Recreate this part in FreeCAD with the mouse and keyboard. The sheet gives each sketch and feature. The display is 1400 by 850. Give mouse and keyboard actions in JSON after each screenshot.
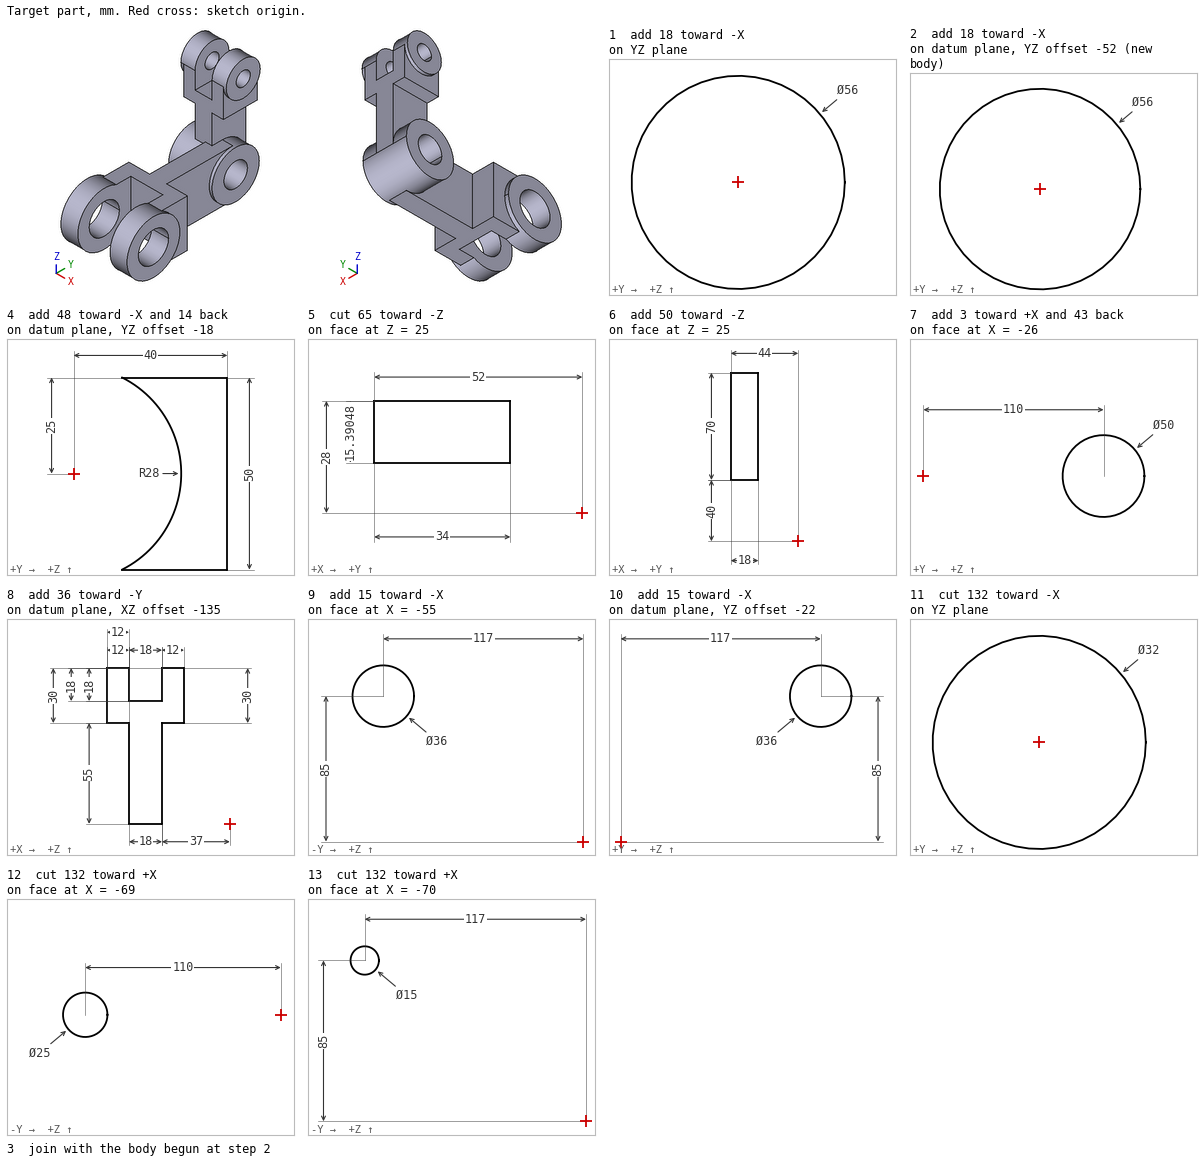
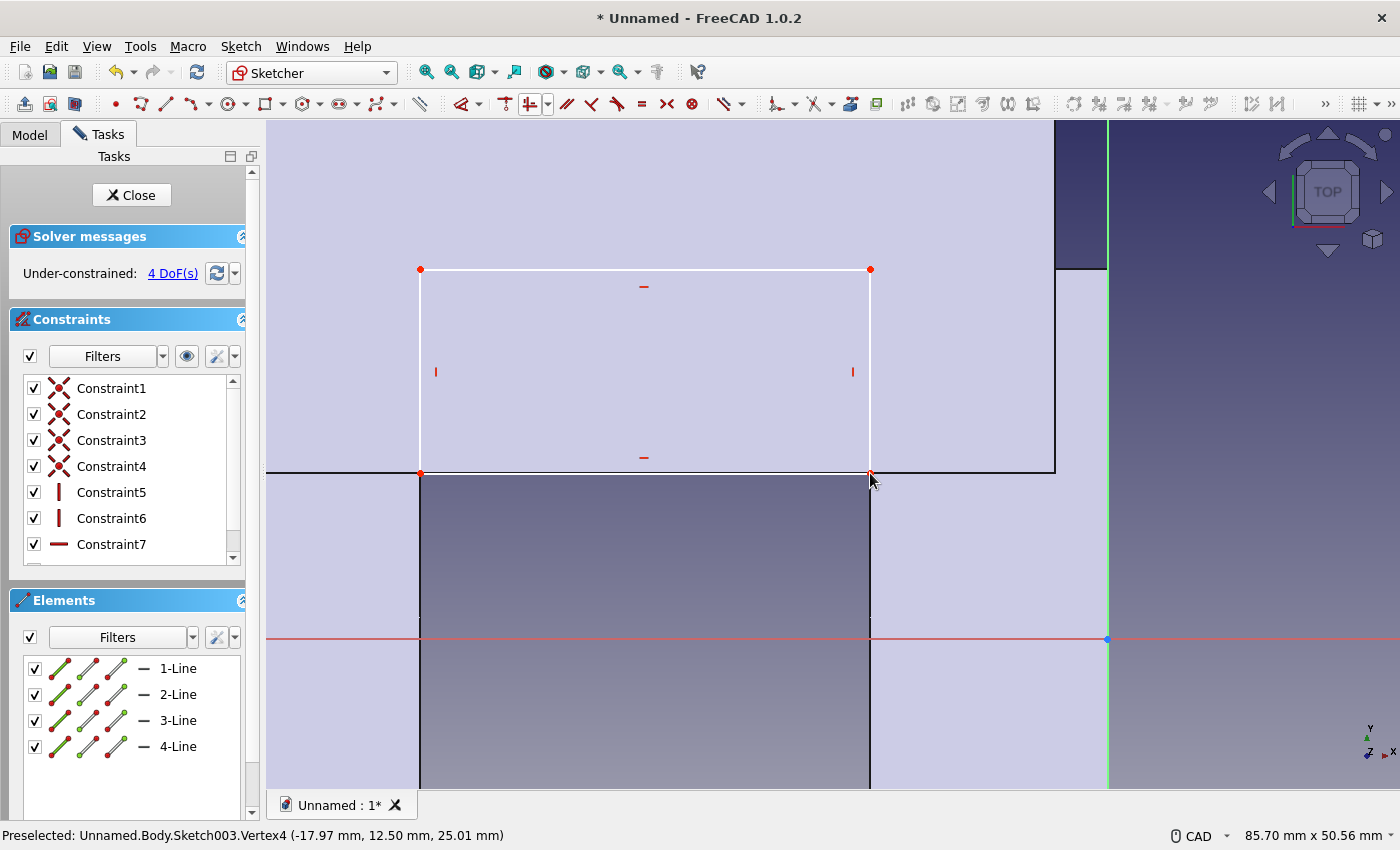
{"action": "left_click", "coordinate": [555, 474]}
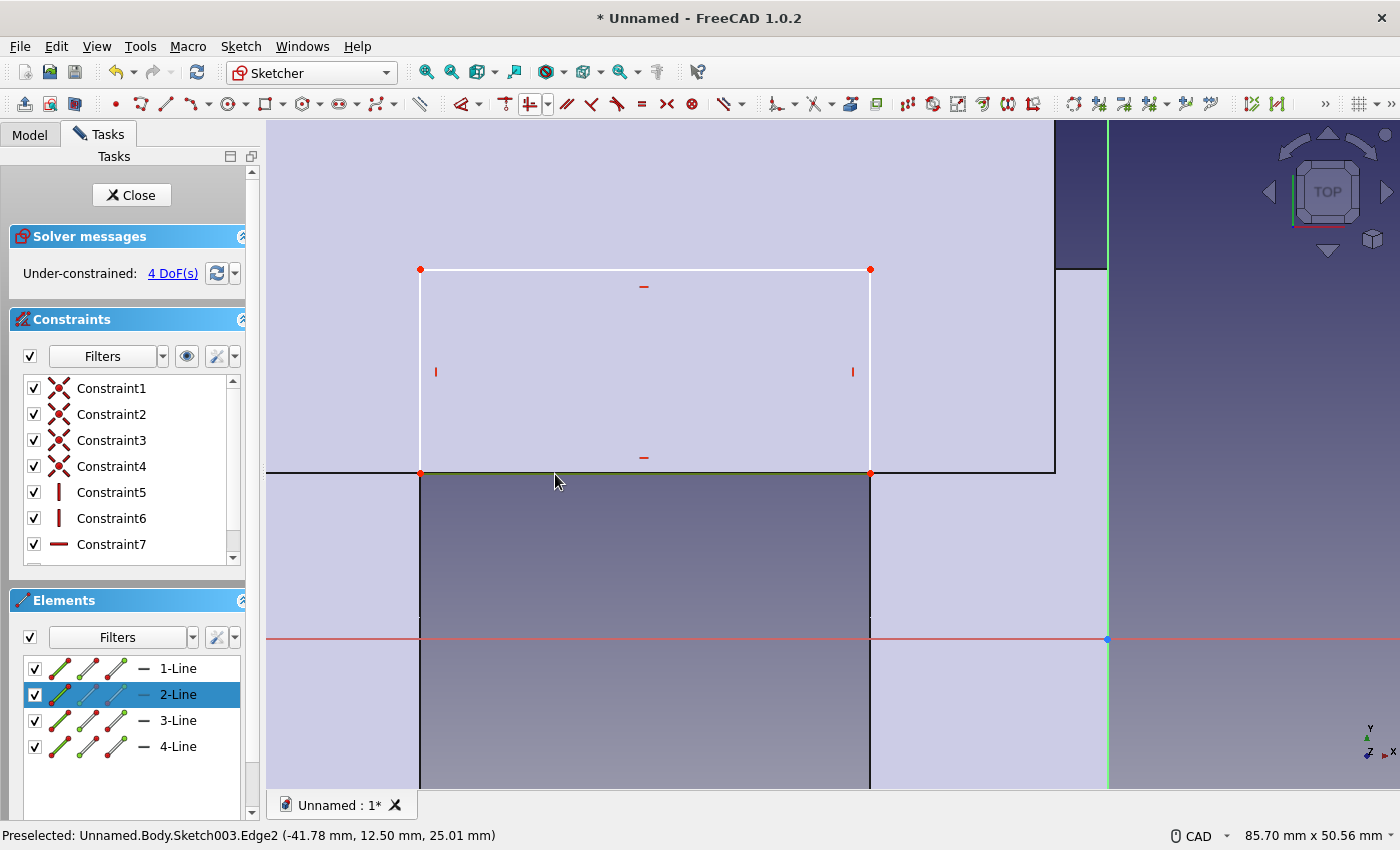
{"action": "key", "text": "l"}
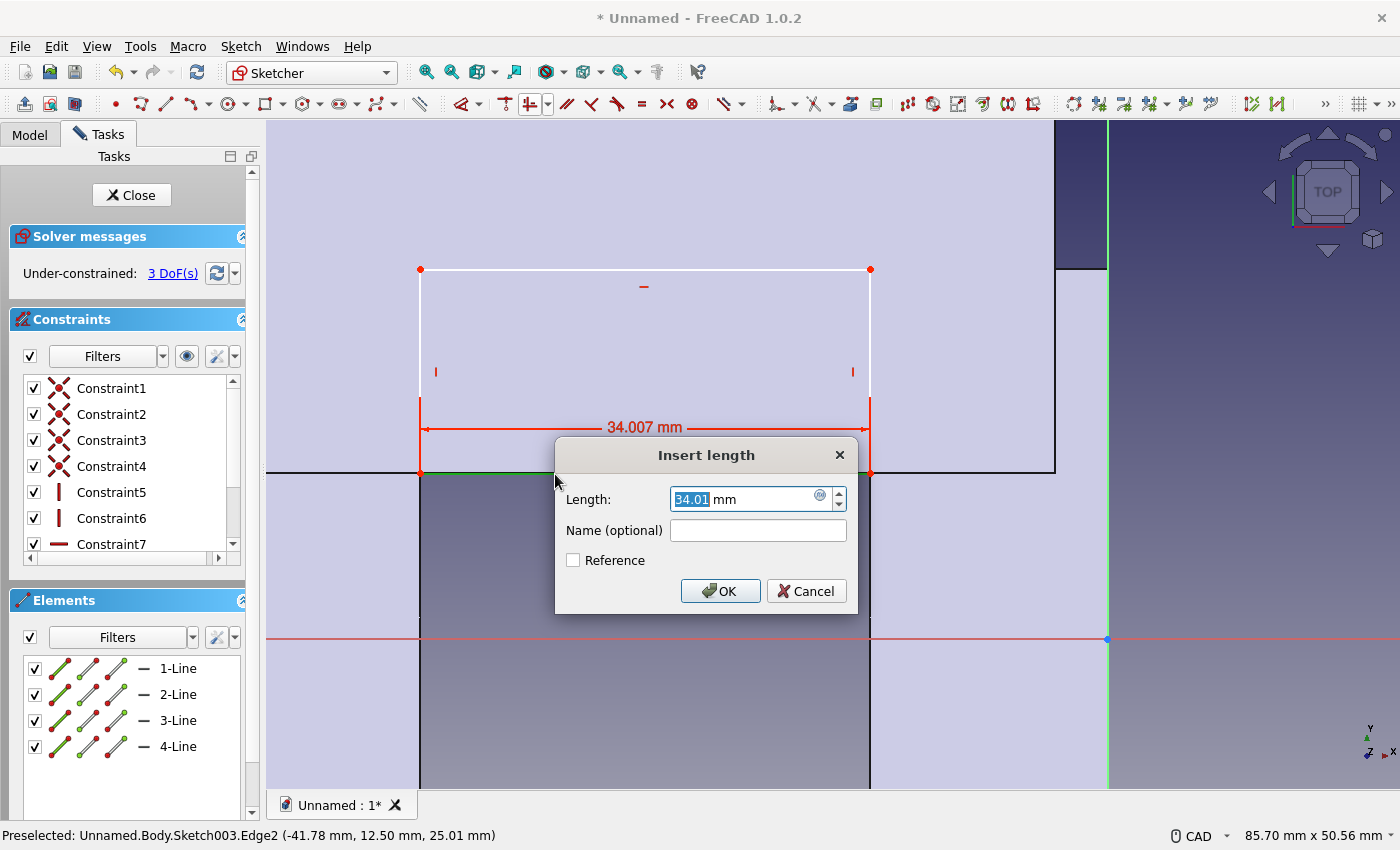
{"action": "type", "text": "34"}
{"action": "key", "text": "Return"}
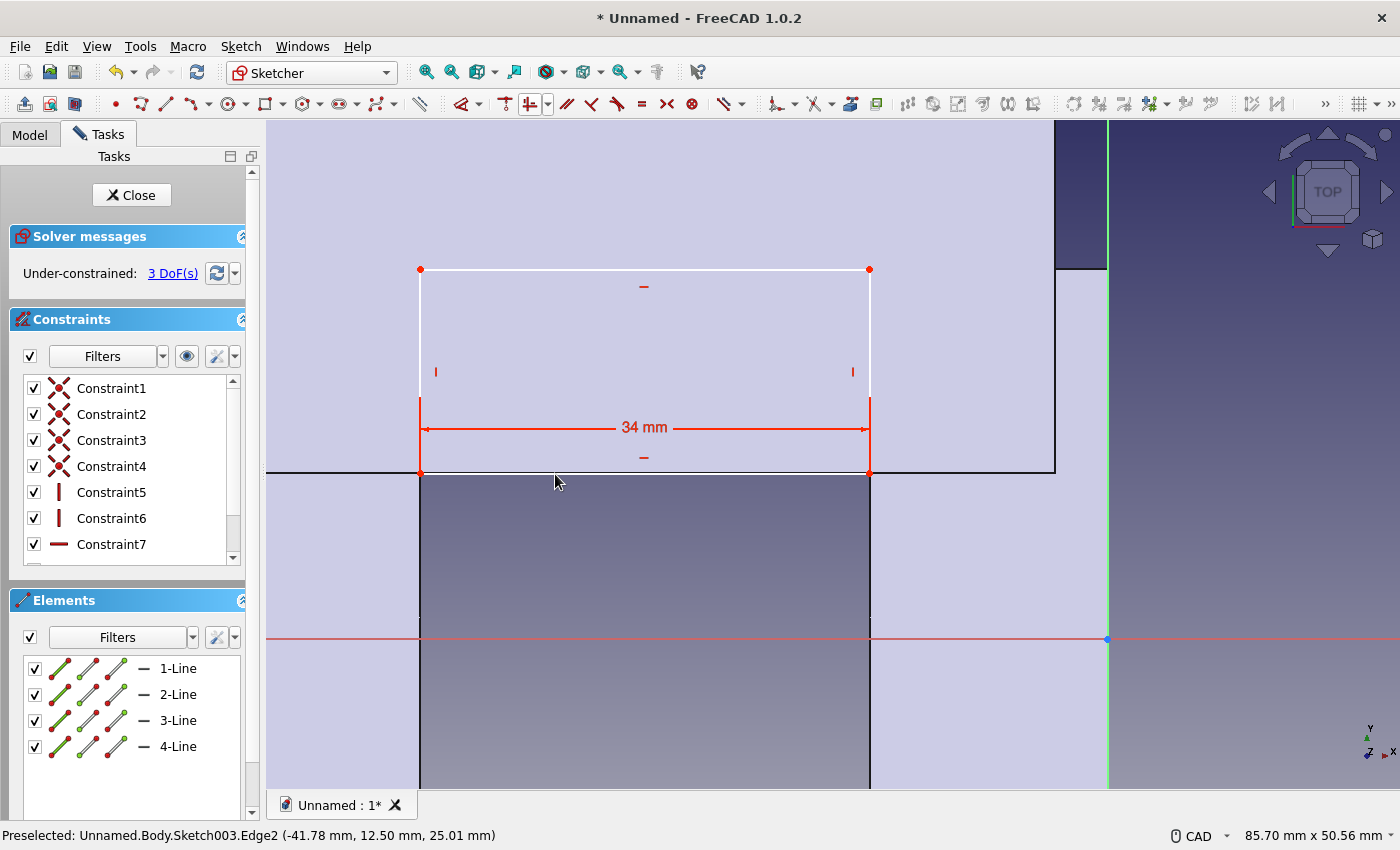
{"action": "left_click", "coordinate": [420, 270]}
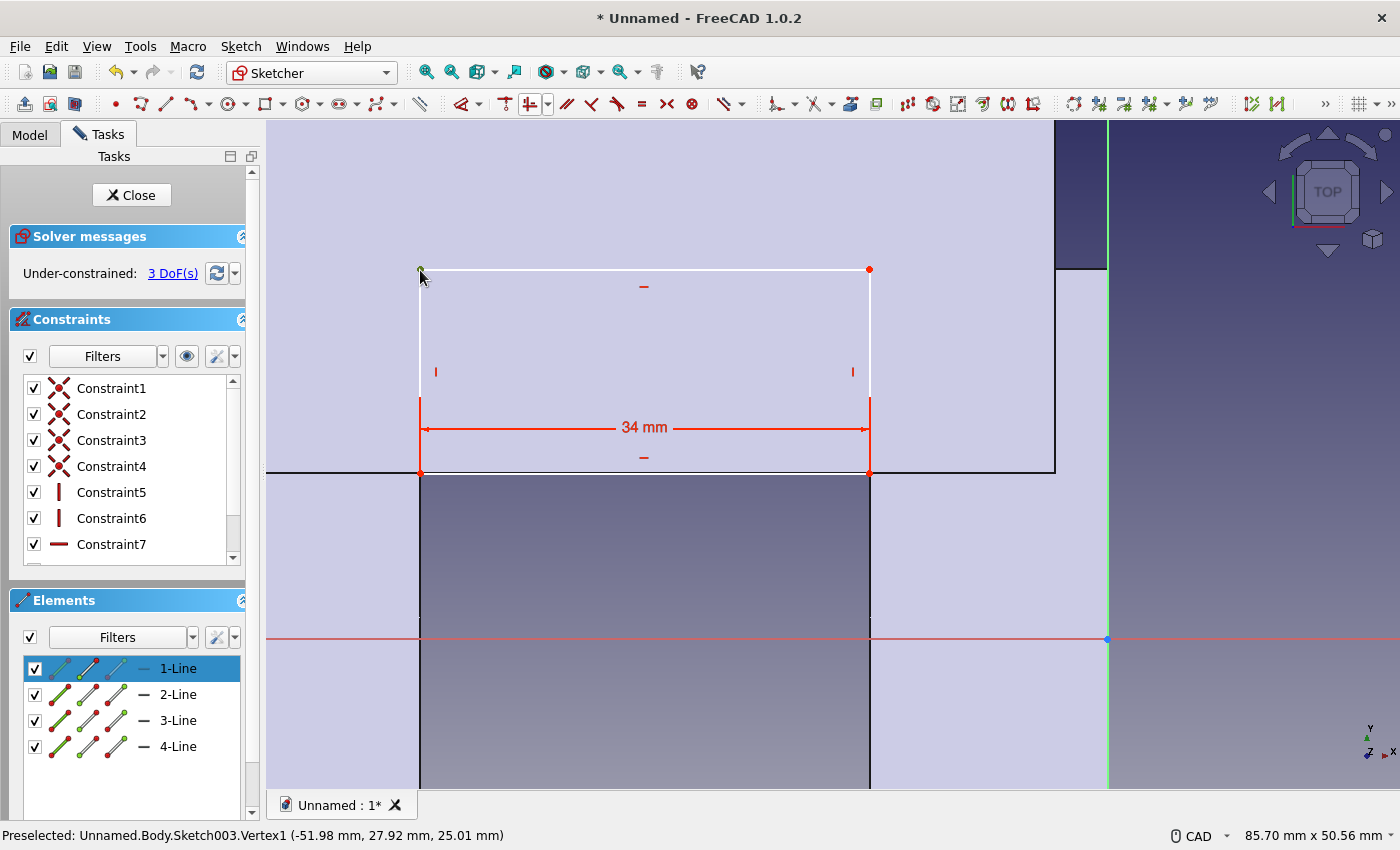
{"action": "key", "text": "l"}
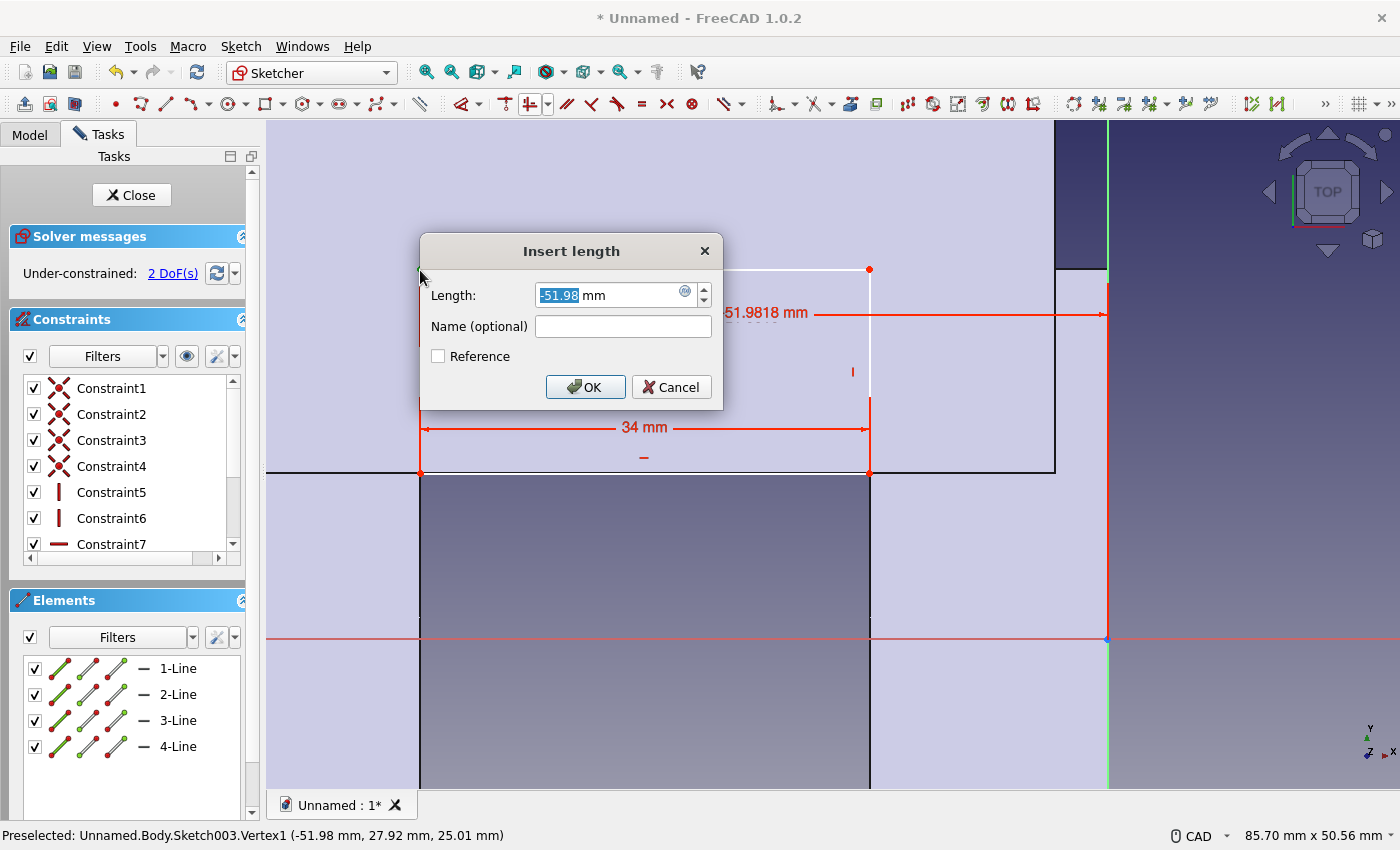
{"action": "type", "text": "-52"}
{"action": "key", "text": "Return"}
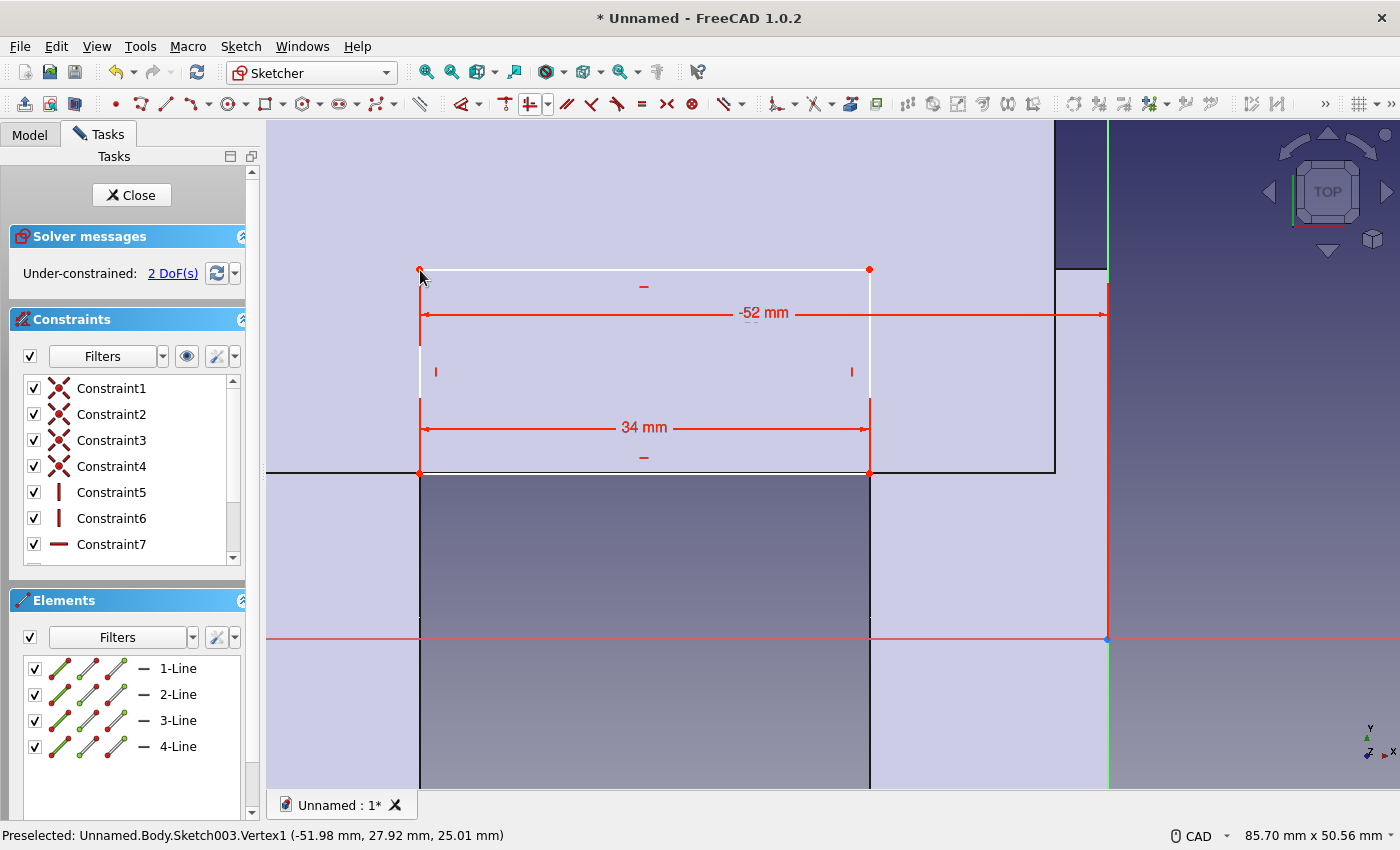
{"action": "left_click", "coordinate": [420, 270]}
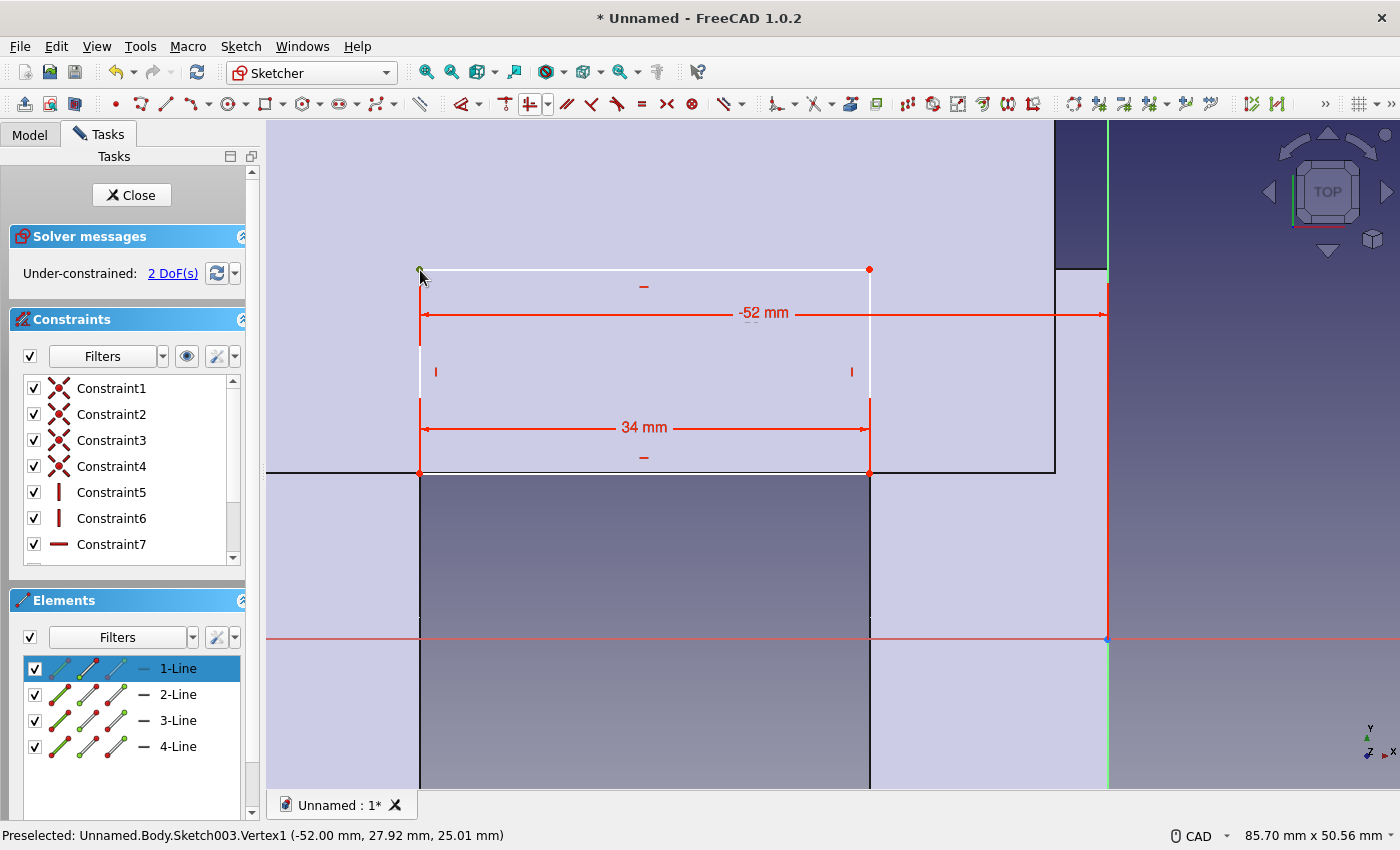
{"action": "key", "text": "i"}